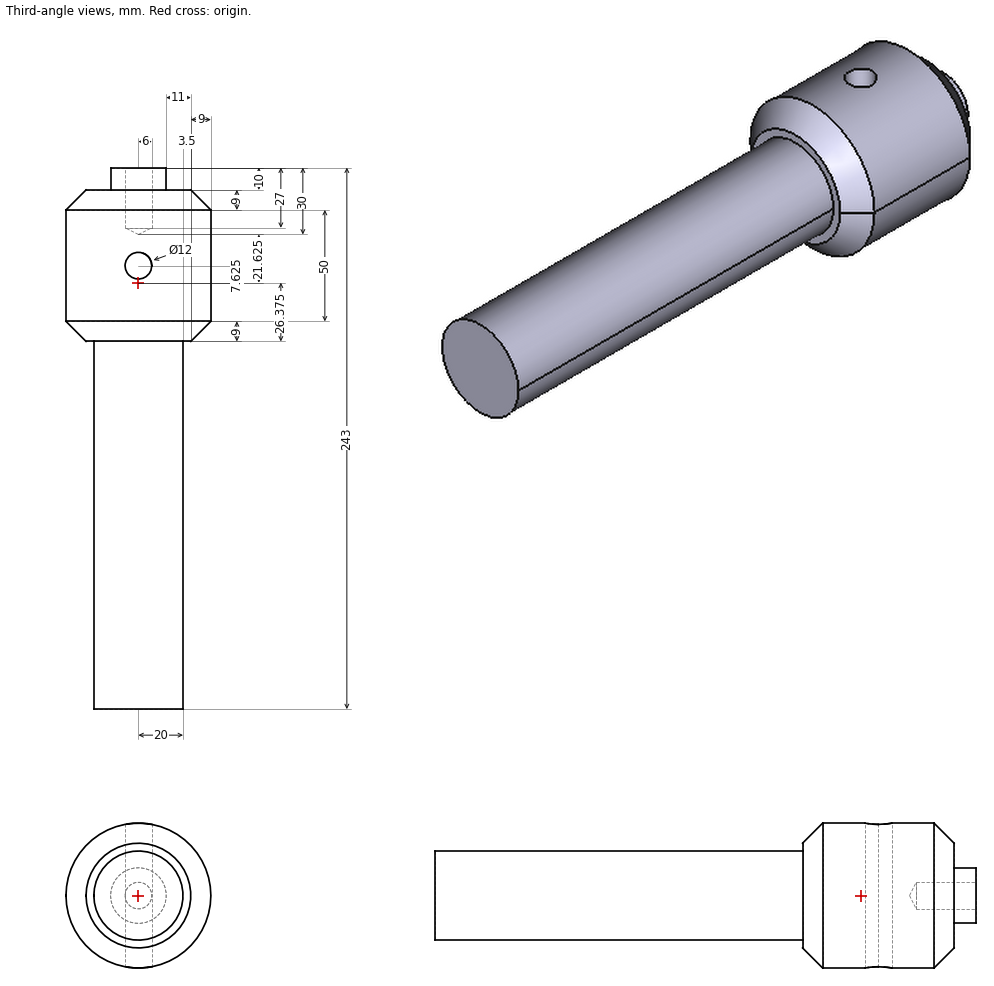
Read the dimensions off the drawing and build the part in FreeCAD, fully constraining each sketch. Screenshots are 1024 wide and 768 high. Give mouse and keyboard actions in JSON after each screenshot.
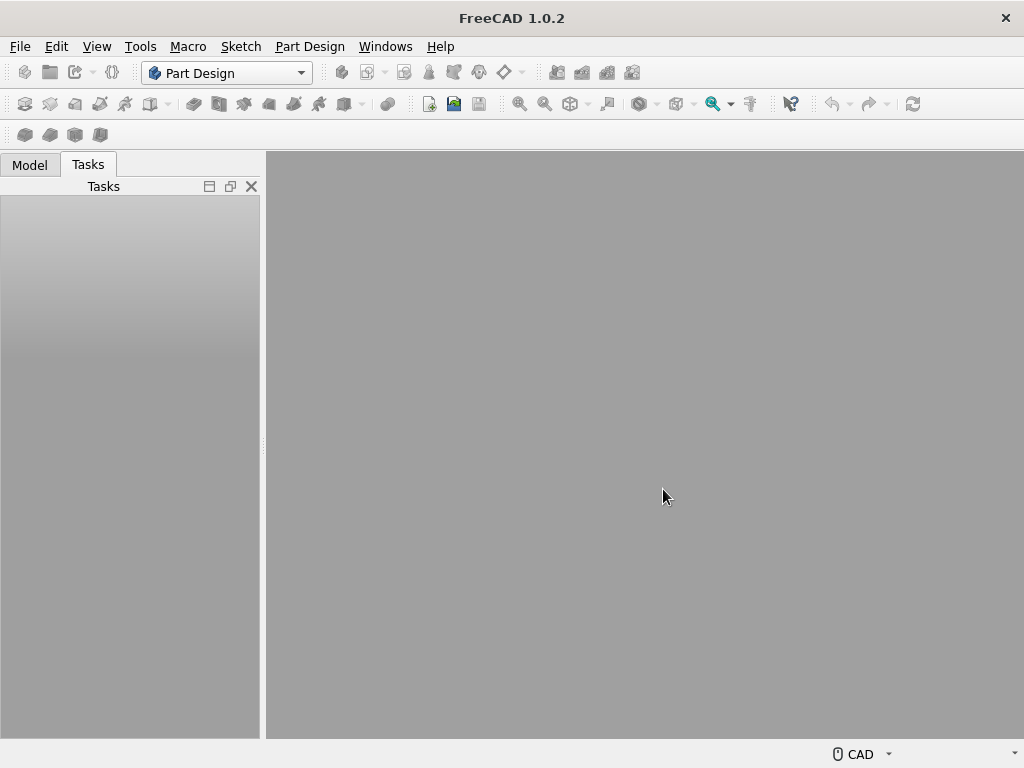
{"action": "left_click", "coordinate": [429, 104]}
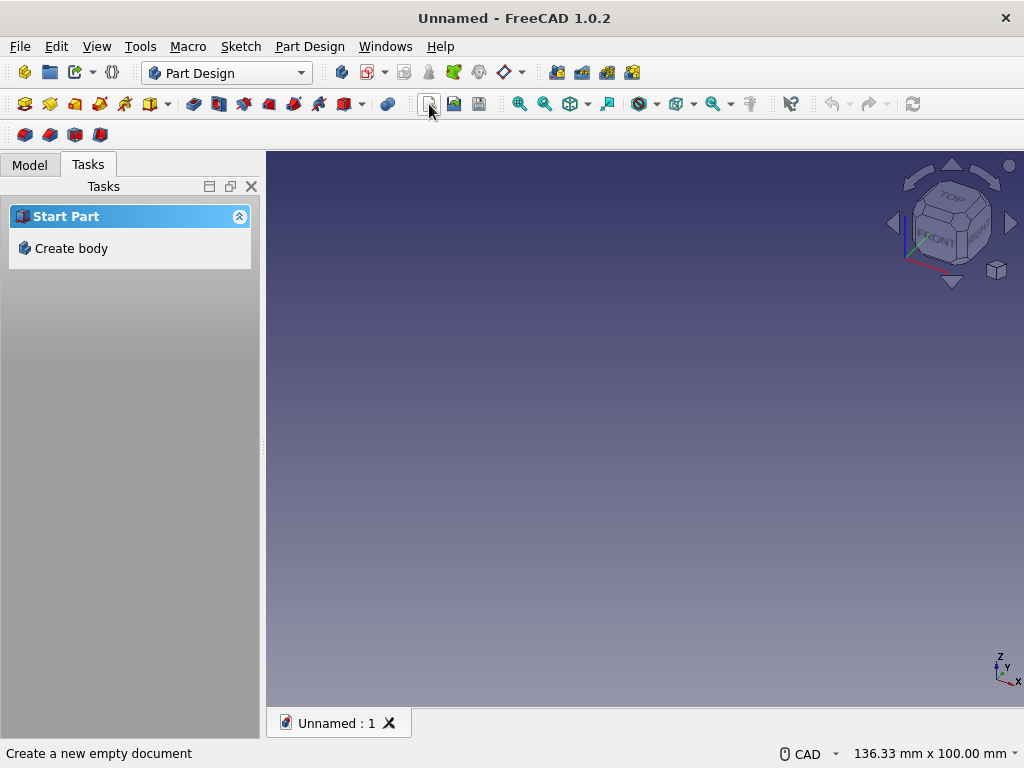
{"action": "left_click", "coordinate": [366, 72]}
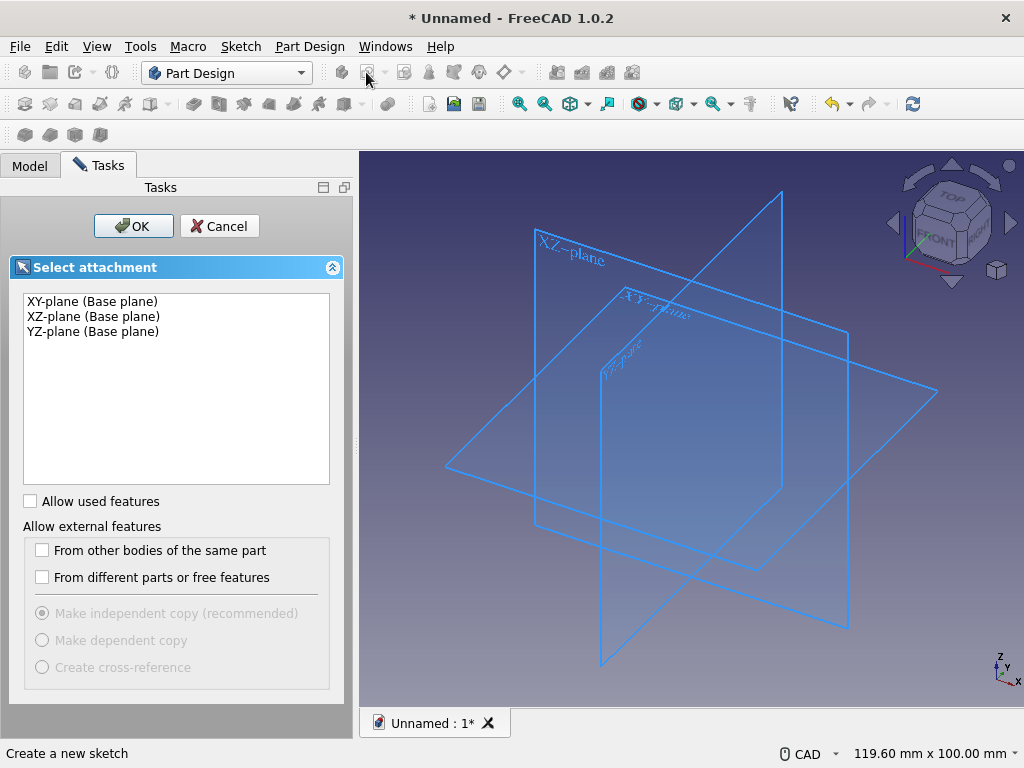
{"action": "left_click", "coordinate": [84, 302]}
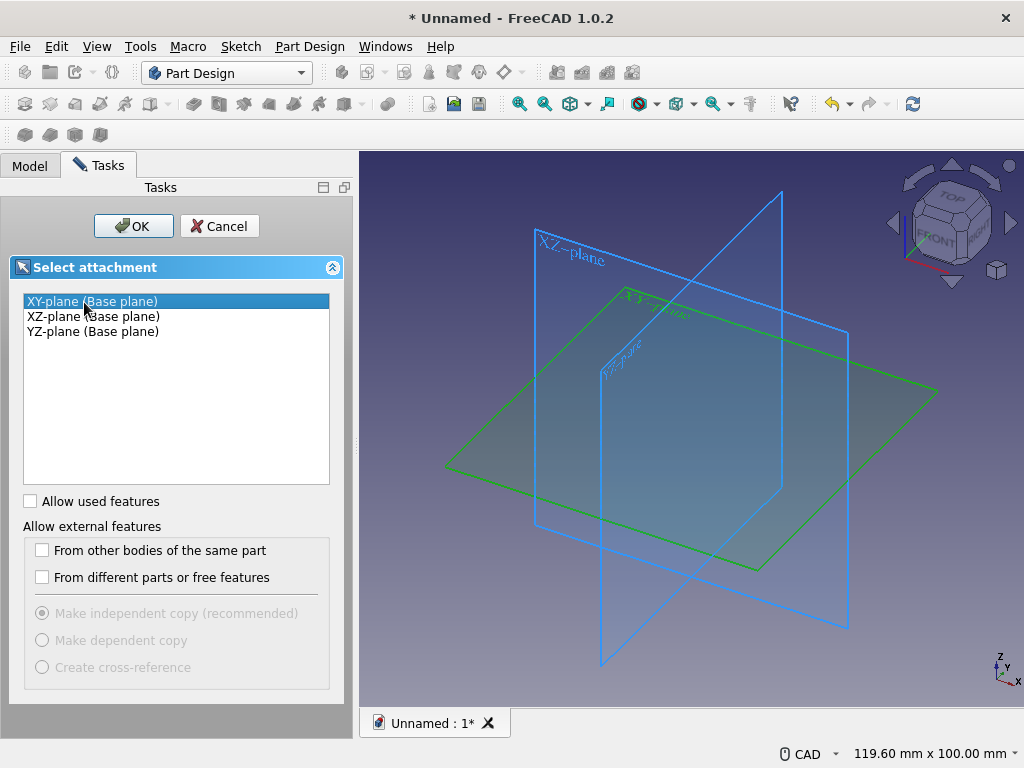
{"action": "left_click", "coordinate": [134, 226]}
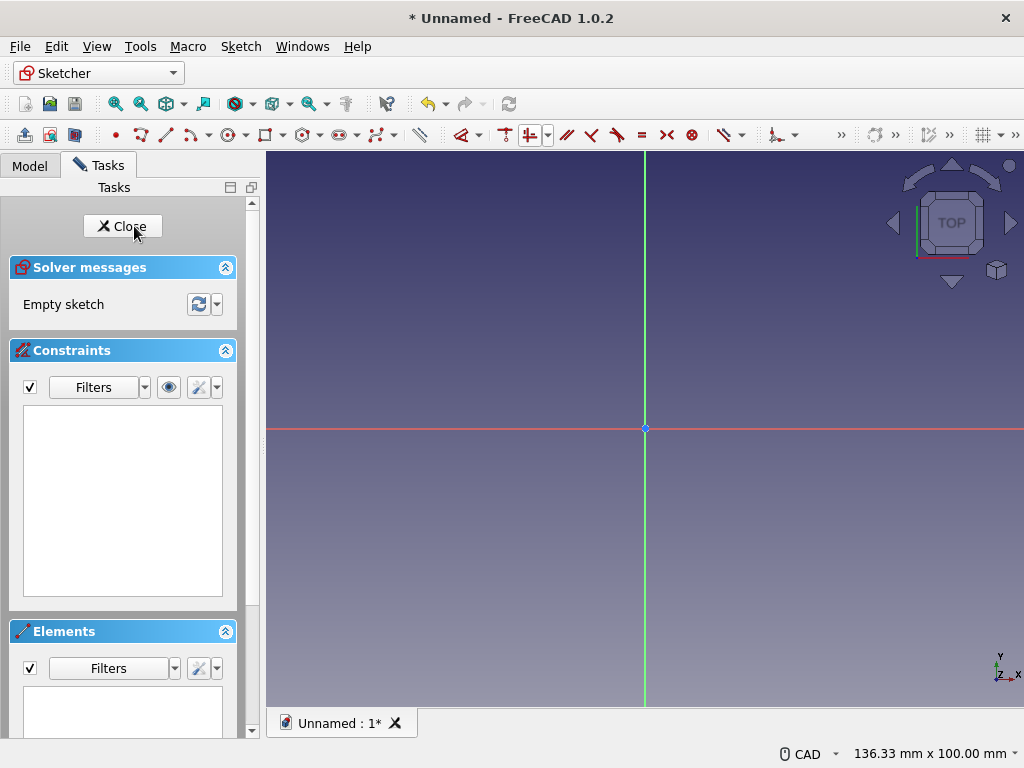
{"action": "scroll", "coordinate": [525, 302], "scroll_direction": "down", "scroll_amount": 7}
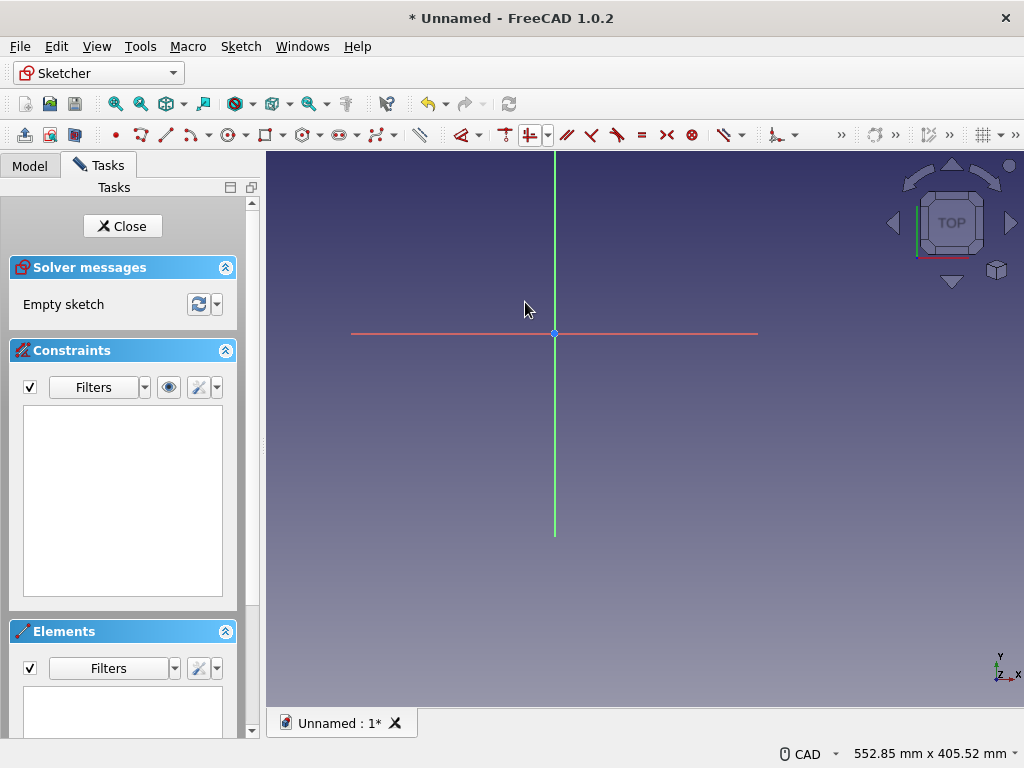
{"action": "left_click", "coordinate": [141, 136]}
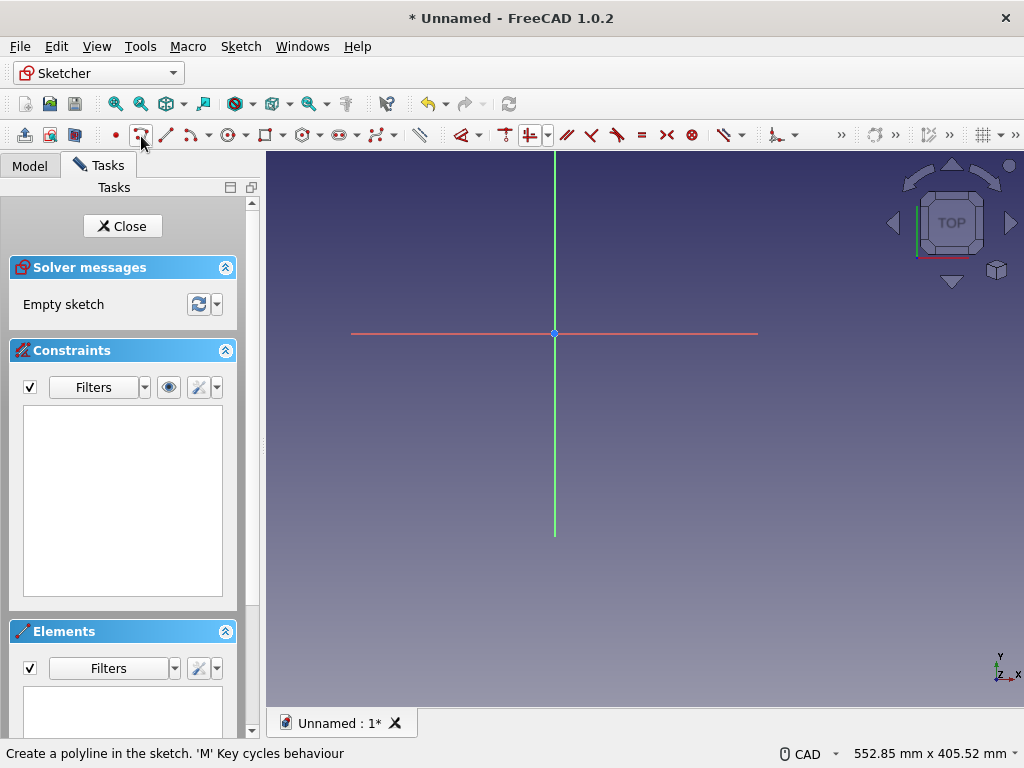
{"action": "left_click", "coordinate": [582, 370]}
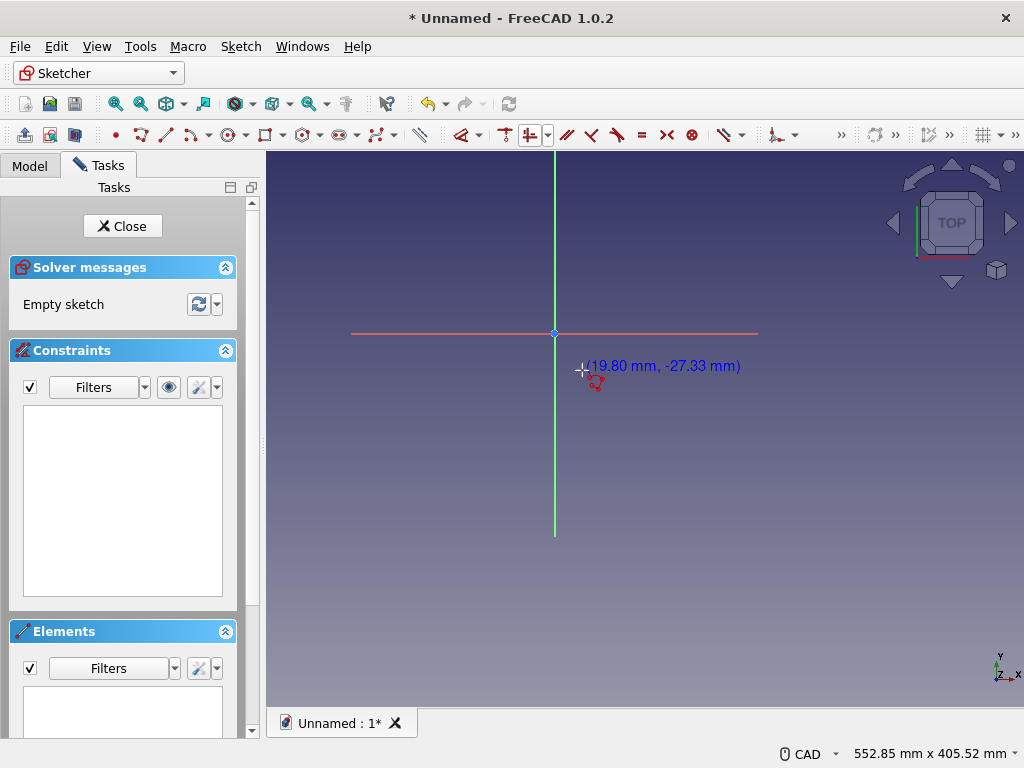
{"action": "scroll", "coordinate": [587, 370], "scroll_direction": "up", "scroll_amount": 6}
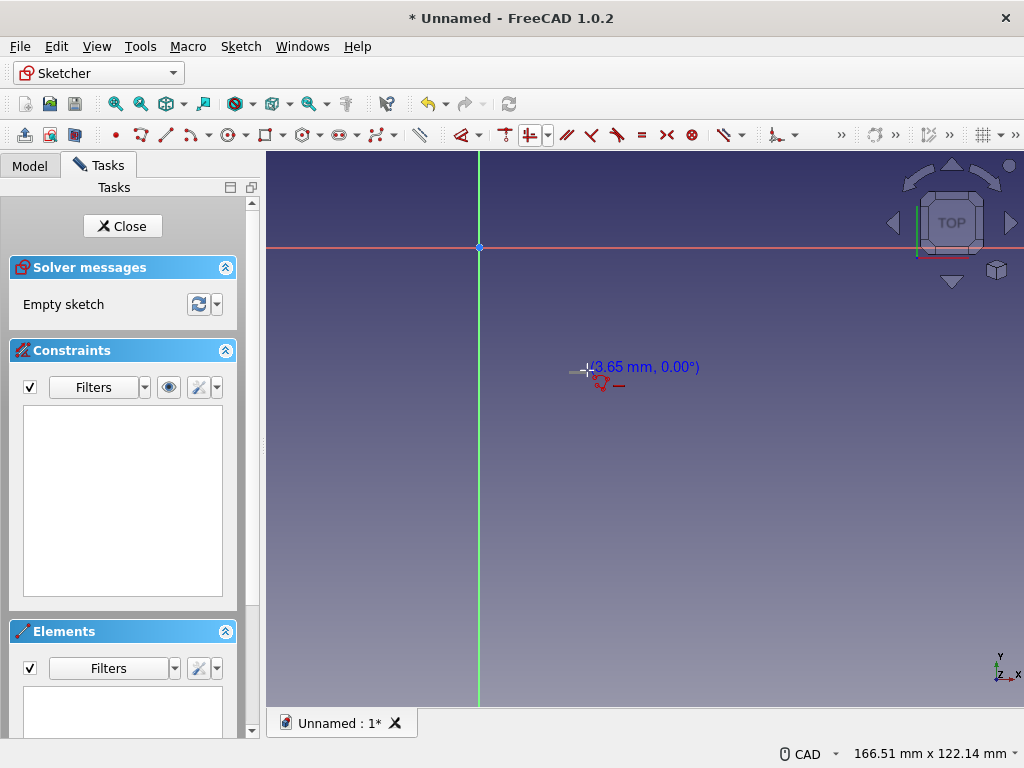
{"action": "left_click", "coordinate": [586, 369]}
{"action": "left_click", "coordinate": [627, 327]}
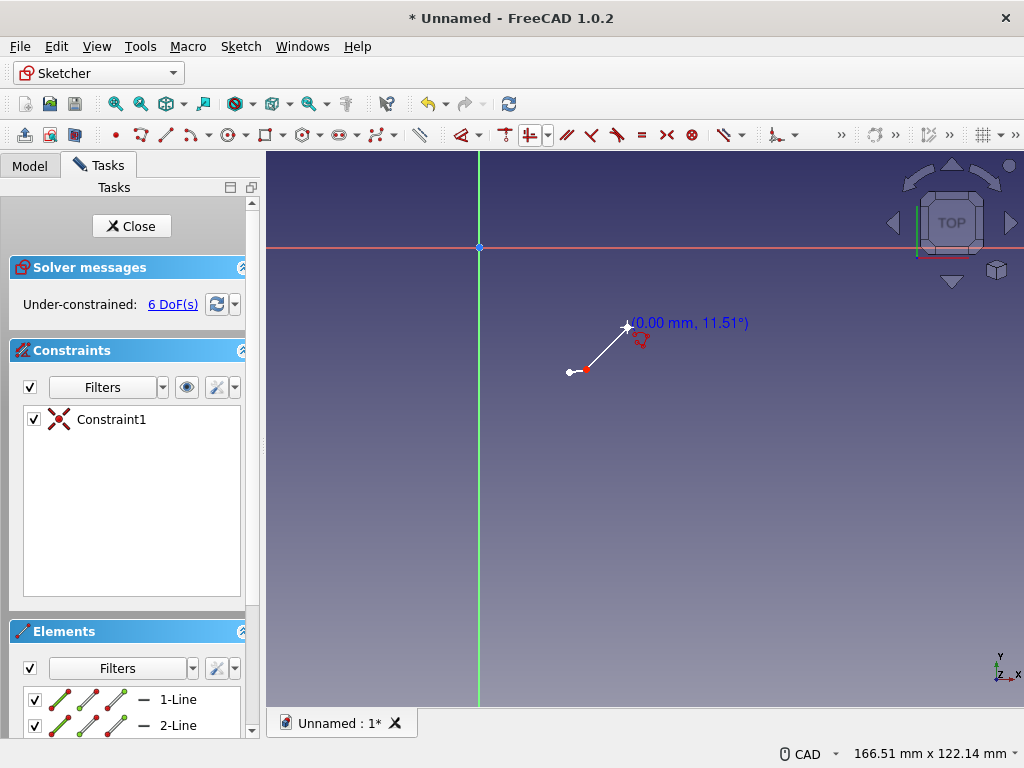
{"action": "scroll", "coordinate": [587, 370], "scroll_direction": "down", "scroll_amount": 6}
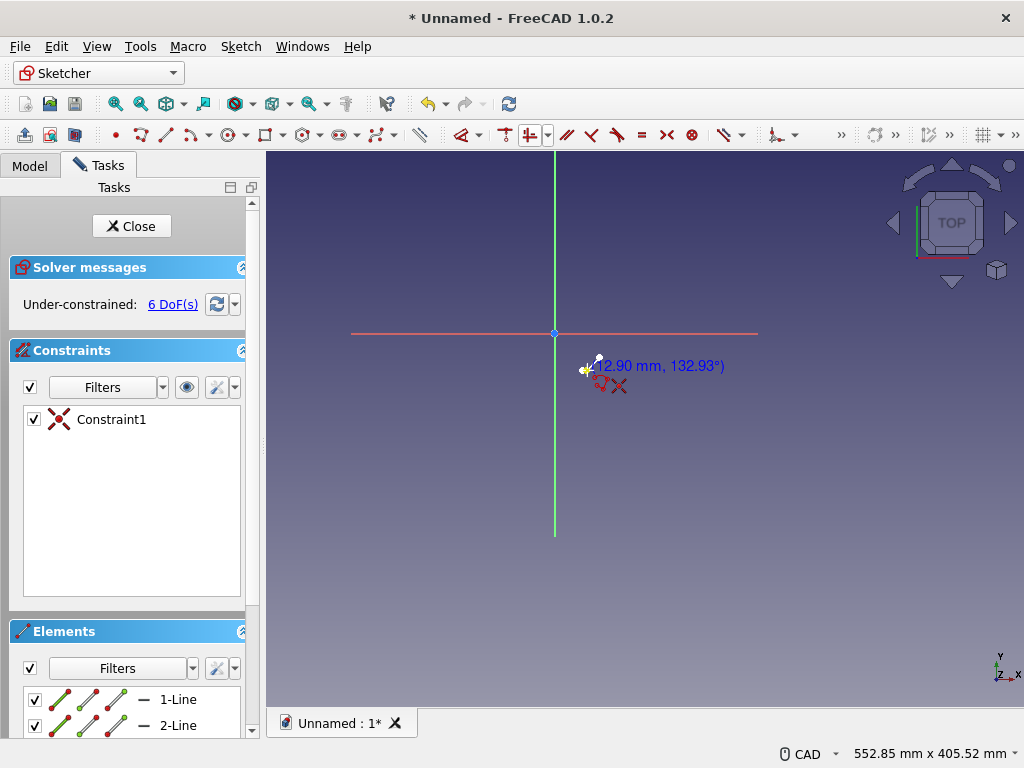
{"action": "left_click", "coordinate": [599, 289]}
{"action": "left_click", "coordinate": [587, 276]}
{"action": "left_click", "coordinate": [572, 276]}
{"action": "left_click", "coordinate": [572, 263]}
{"action": "left_click", "coordinate": [555, 263]}
{"action": "left_click", "coordinate": [564, 596]}
{"action": "left_click", "coordinate": [582, 596]}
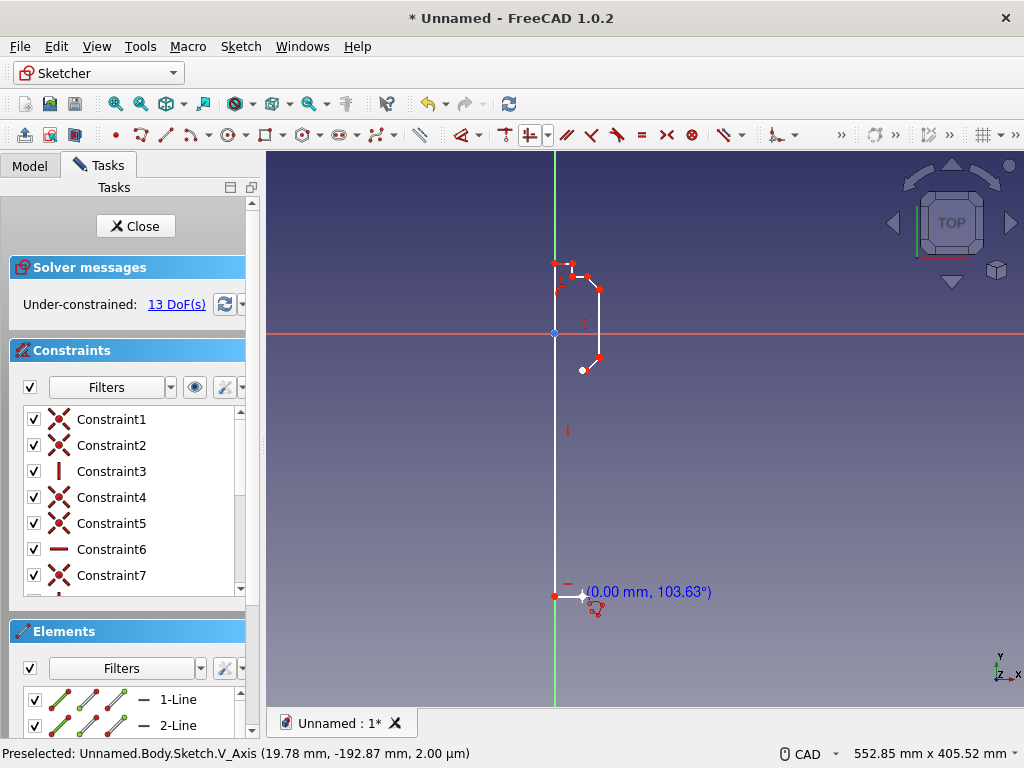
{"action": "scroll", "coordinate": [582, 370], "scroll_direction": "up", "scroll_amount": 10}